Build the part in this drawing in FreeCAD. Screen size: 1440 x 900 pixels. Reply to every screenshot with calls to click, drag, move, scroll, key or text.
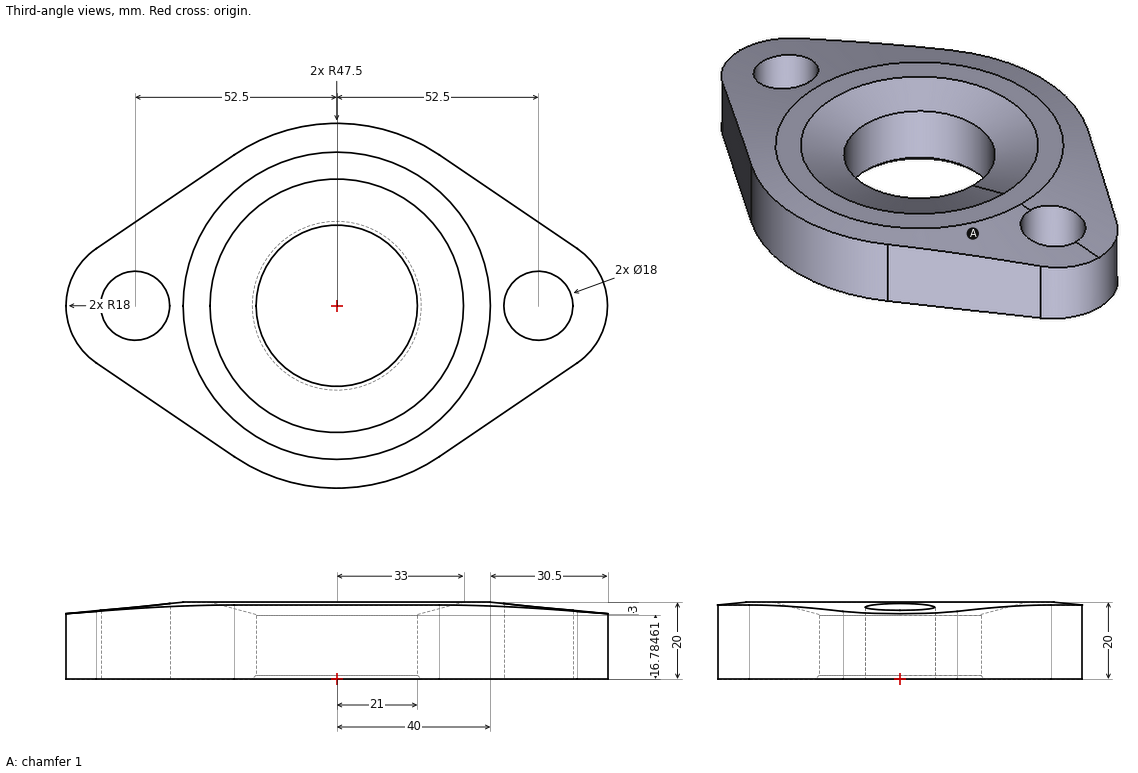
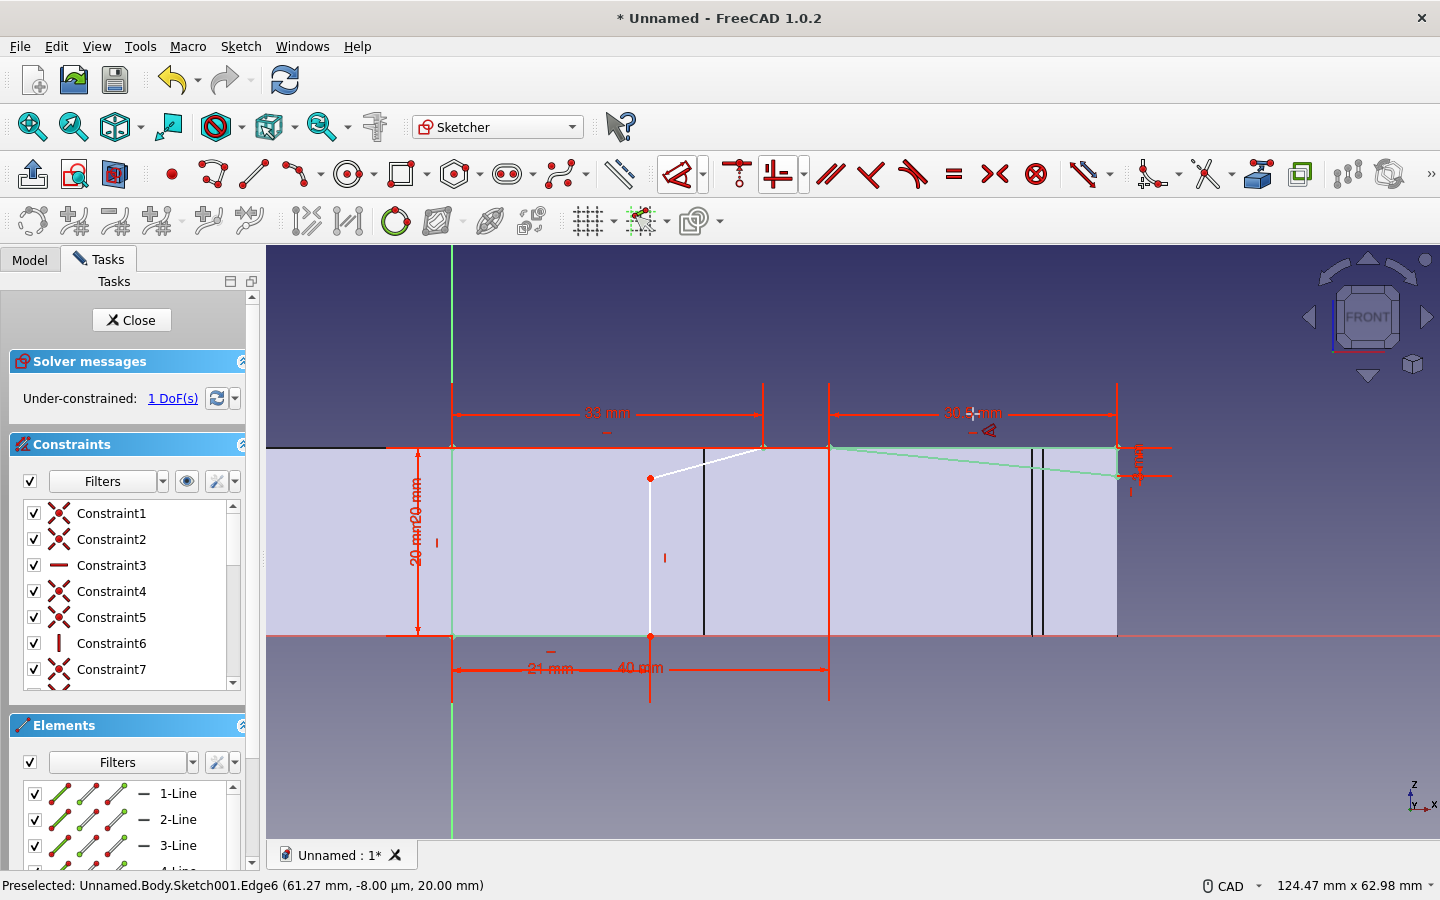
click(650, 526)
click(616, 558)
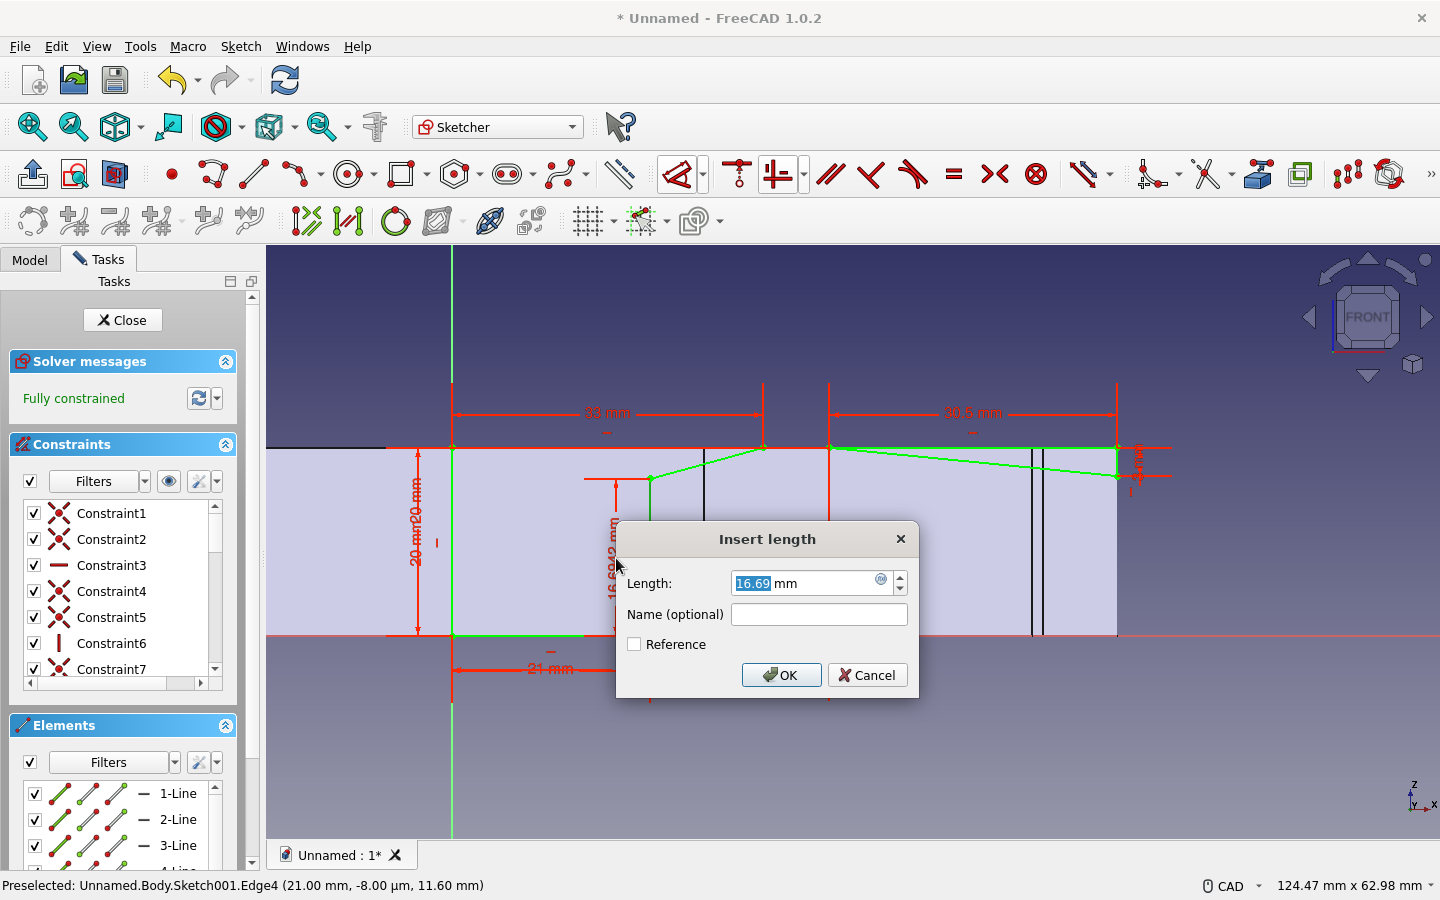
text(16.78461)
key(Return)
key(Escape)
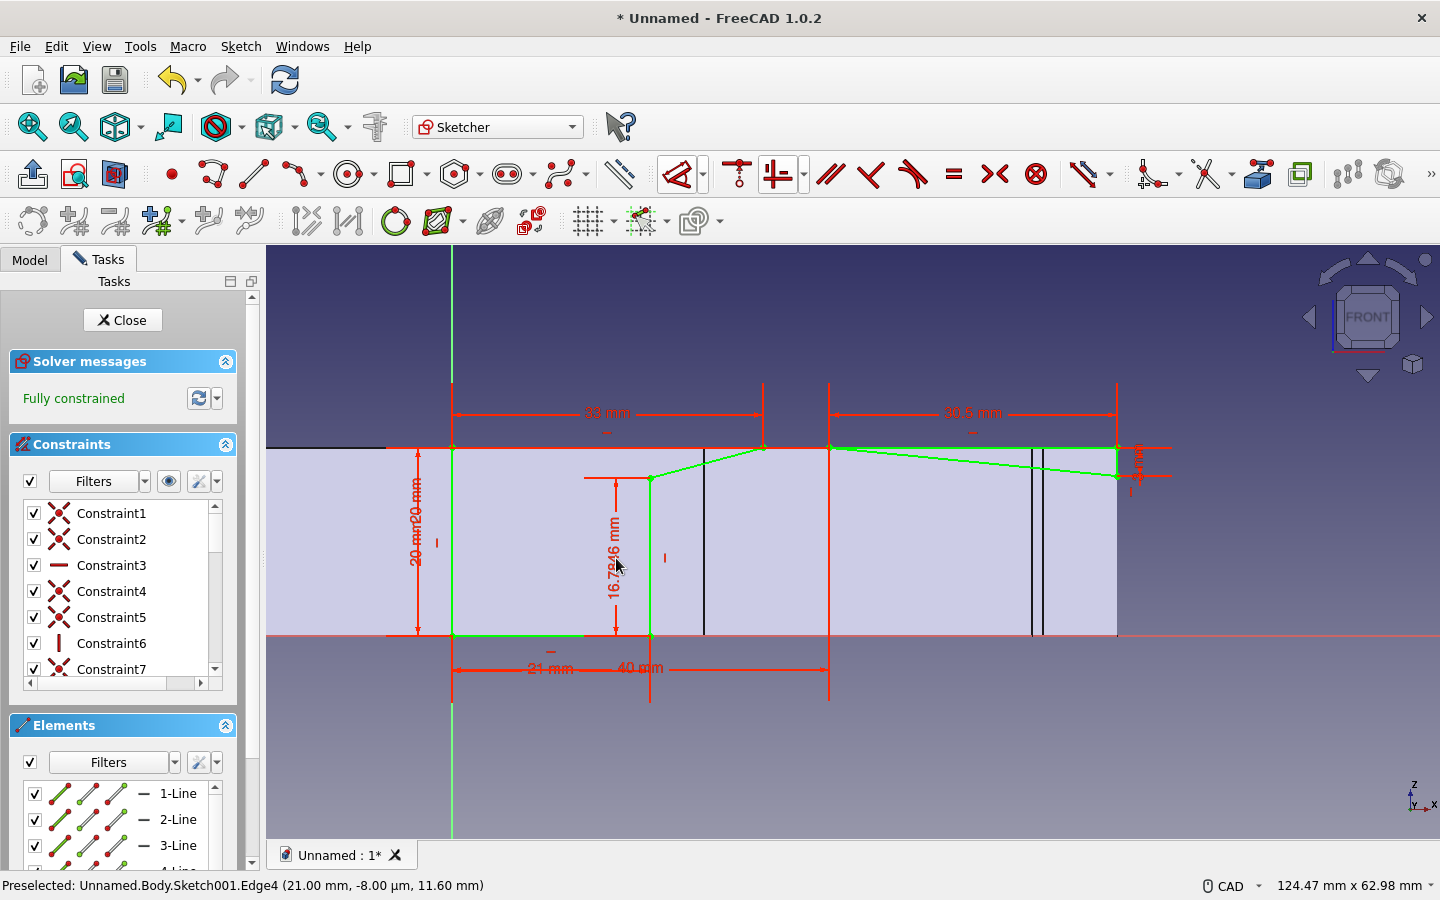
click(123, 320)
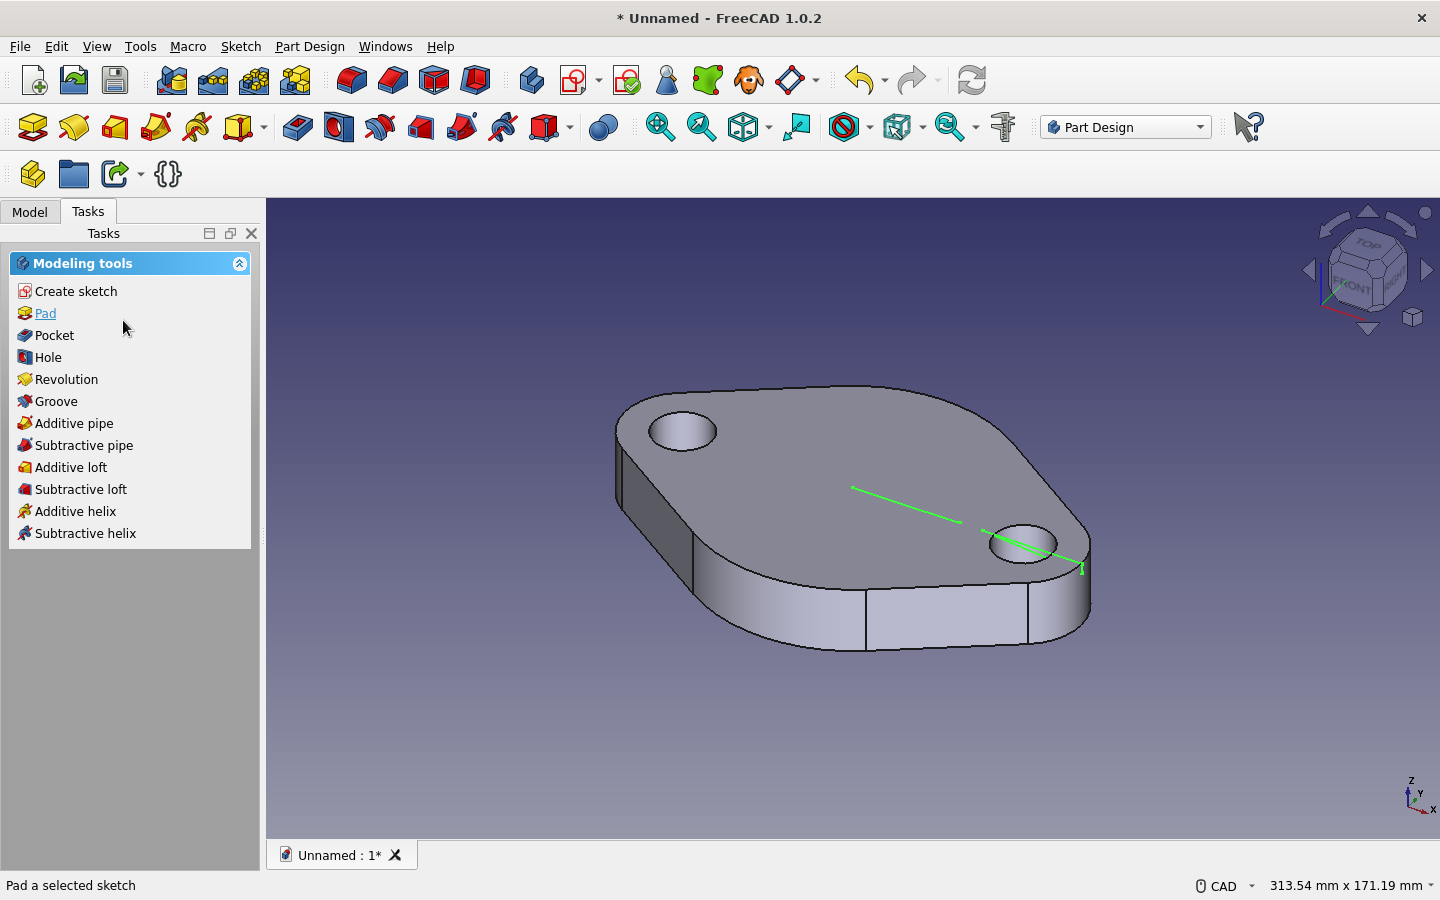
click(380, 128)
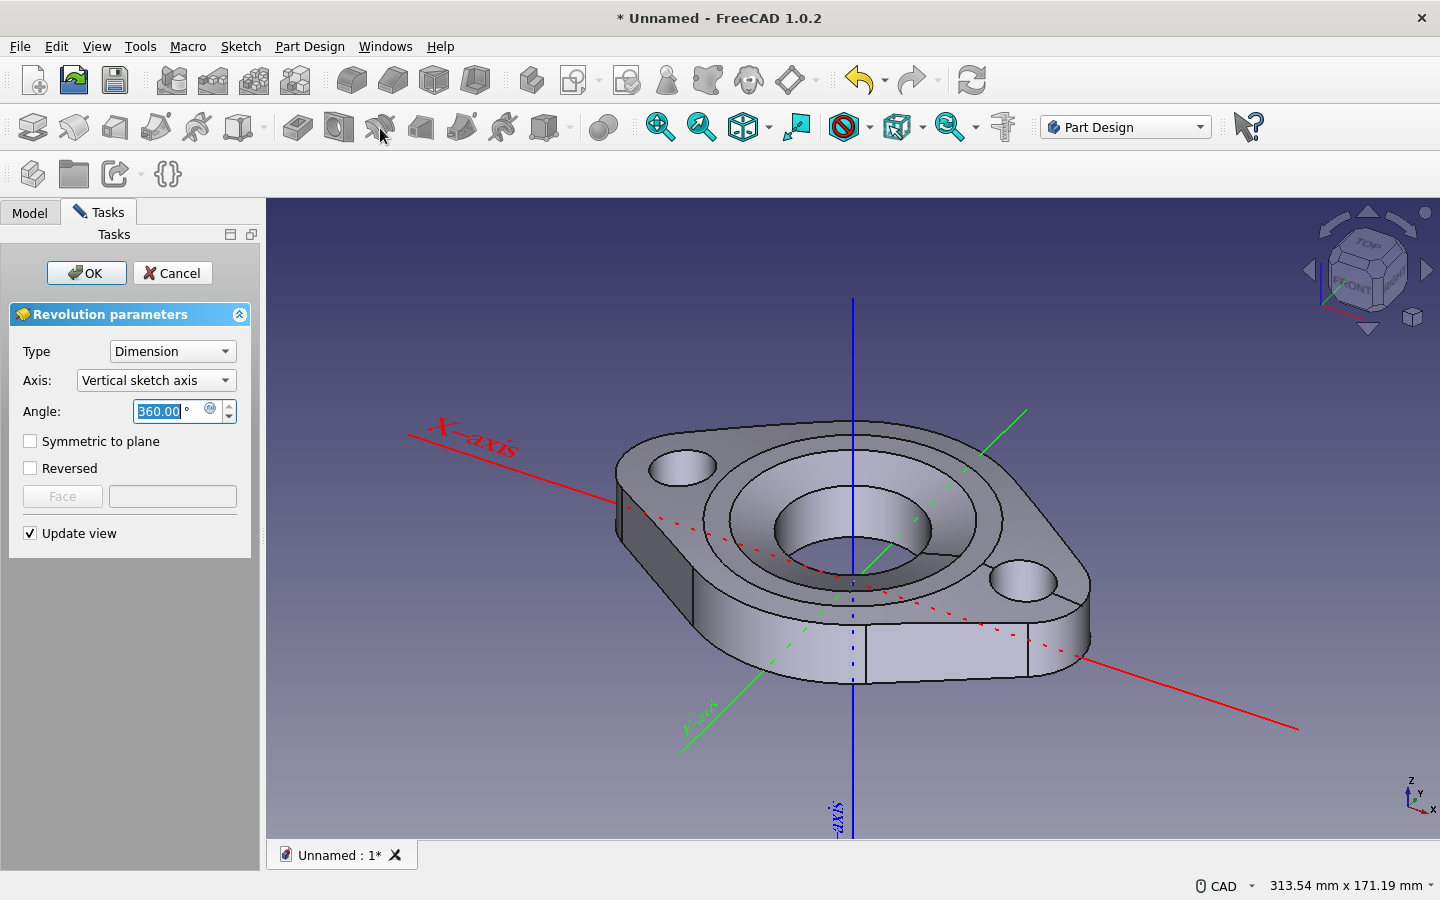
click(87, 273)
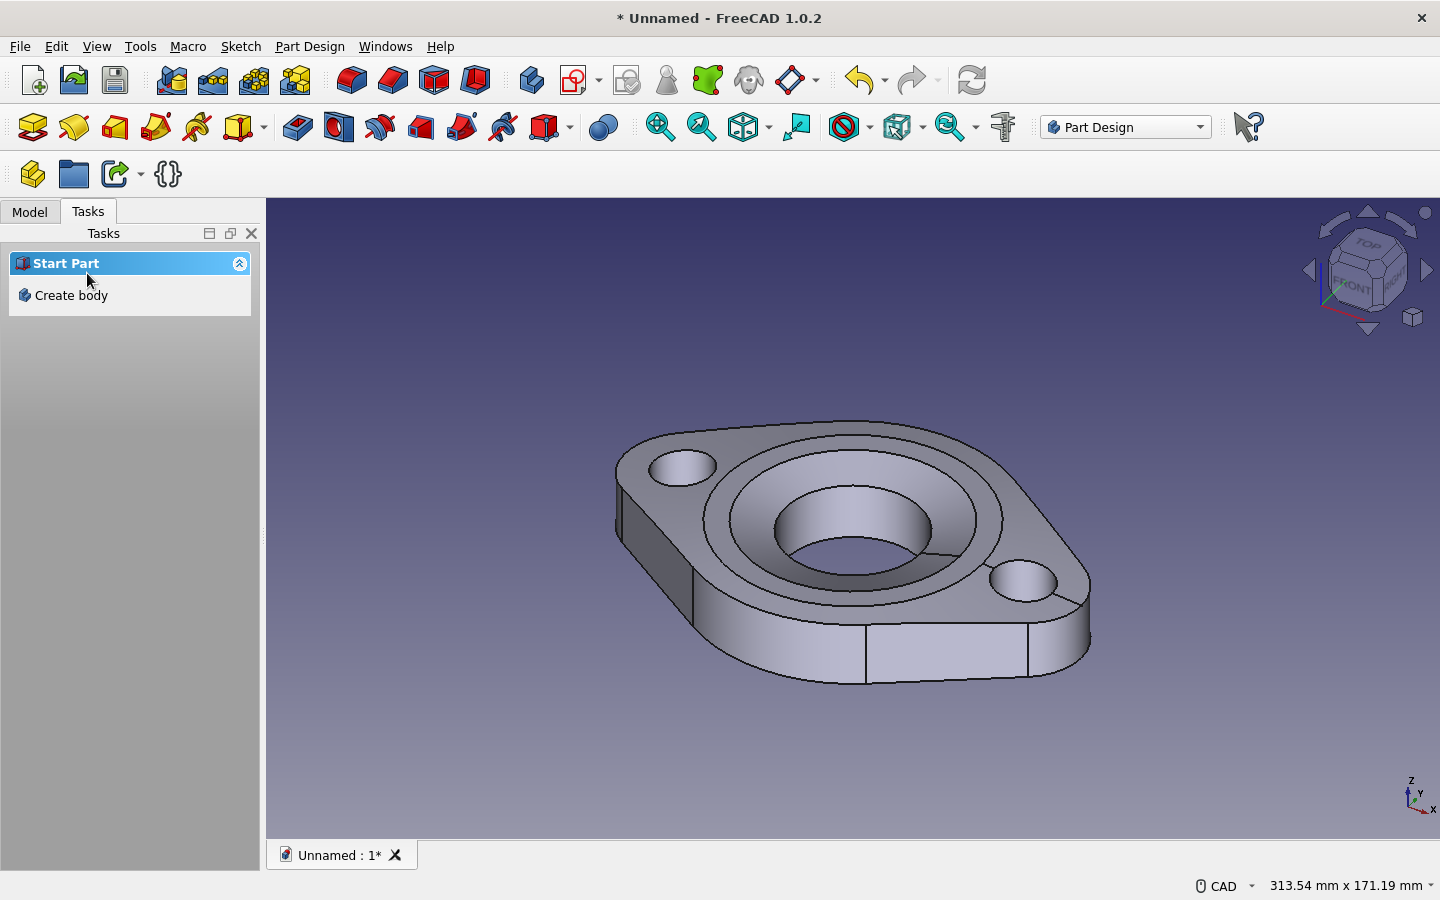
key(0)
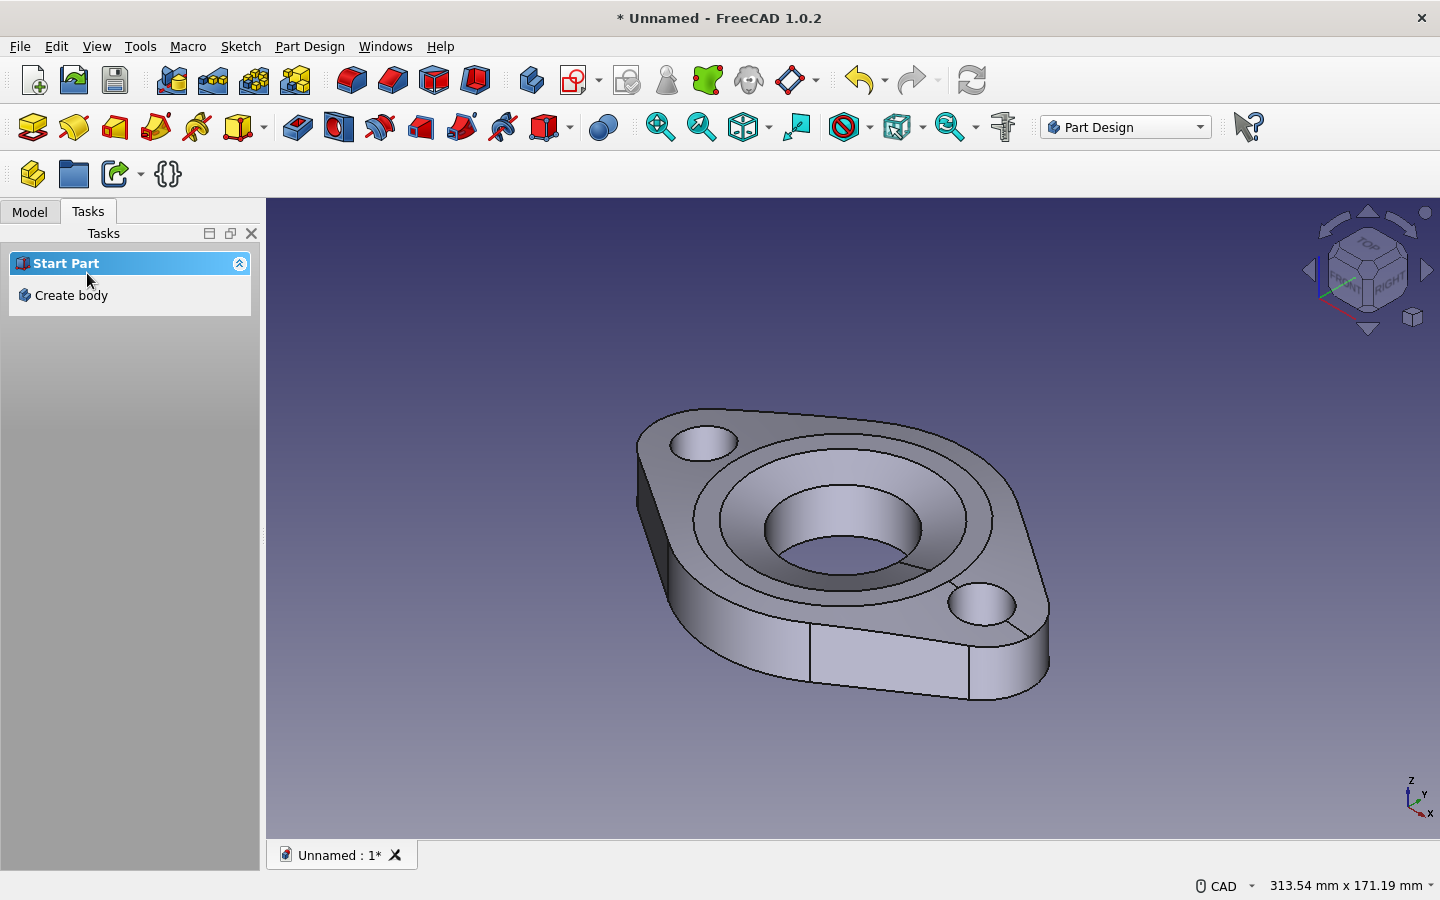
key(2)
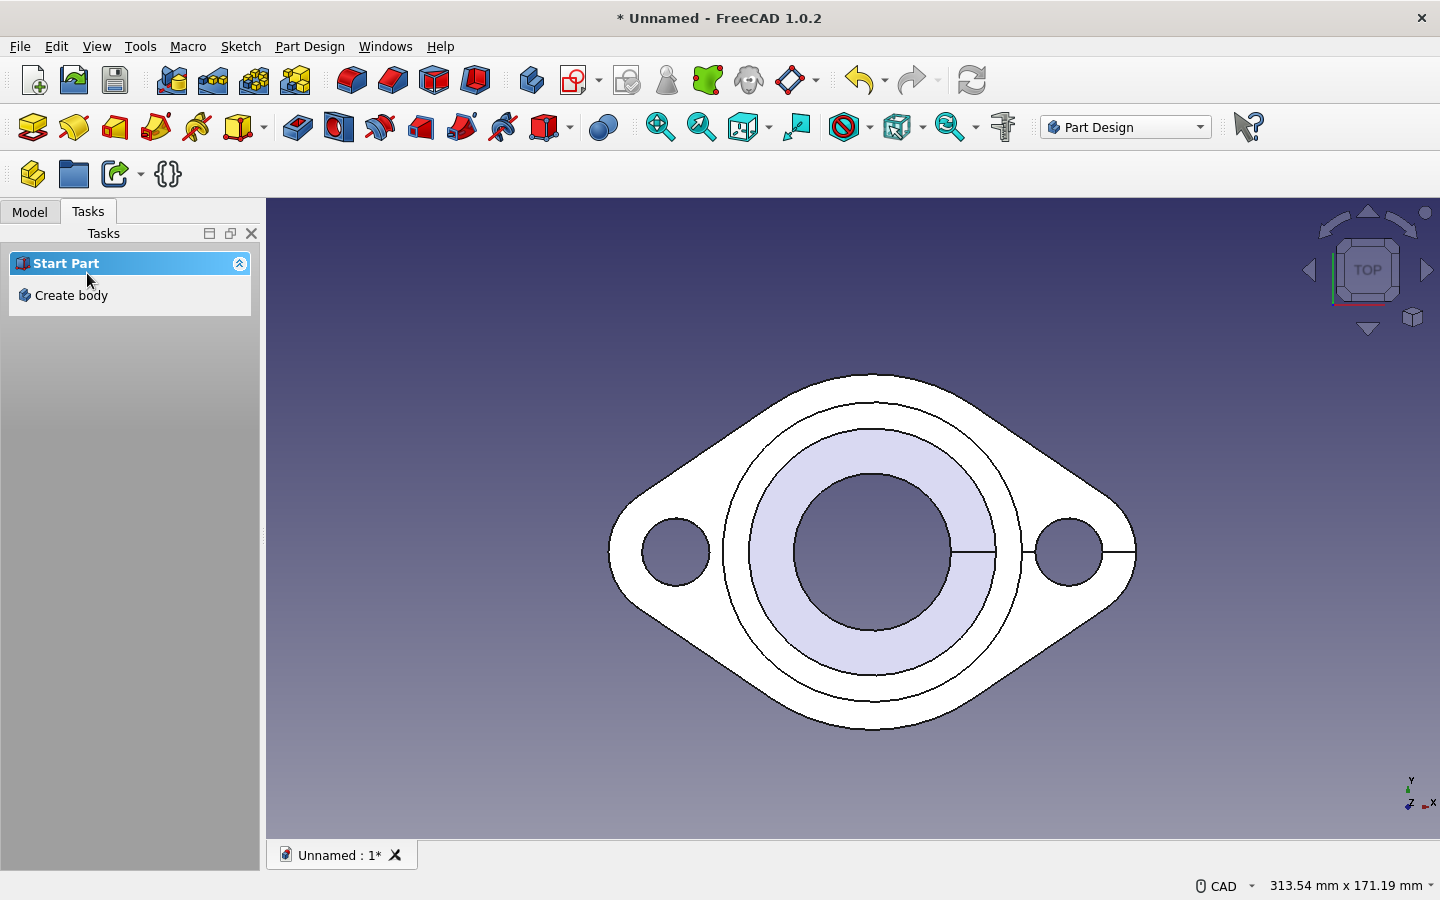
key(1)